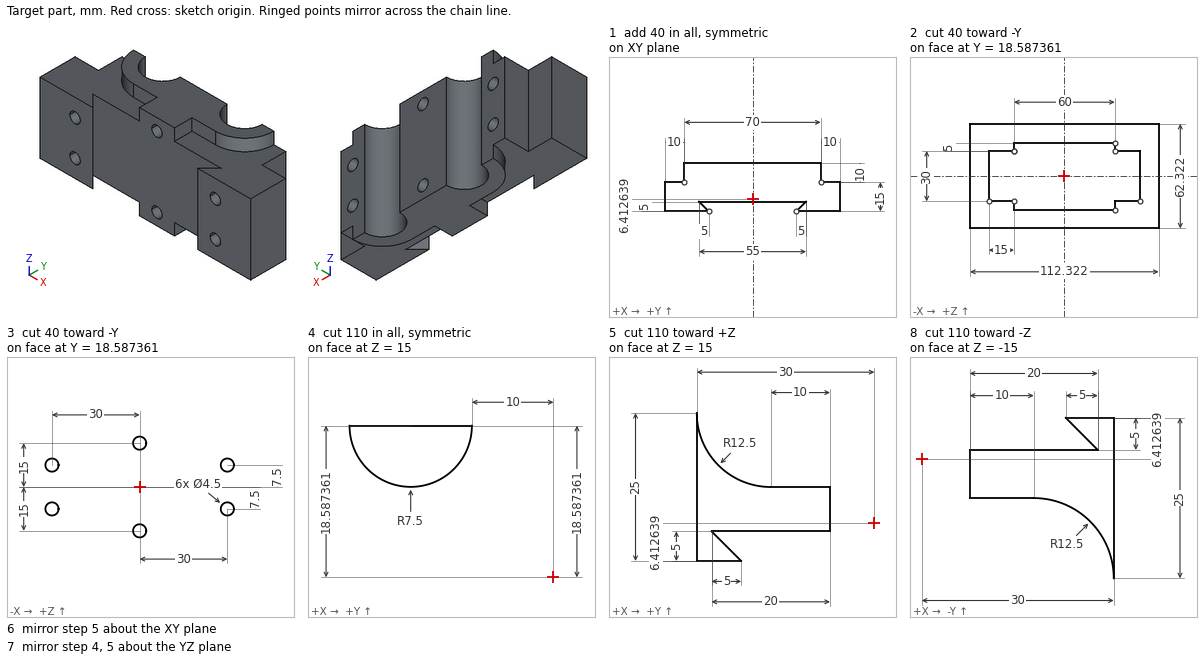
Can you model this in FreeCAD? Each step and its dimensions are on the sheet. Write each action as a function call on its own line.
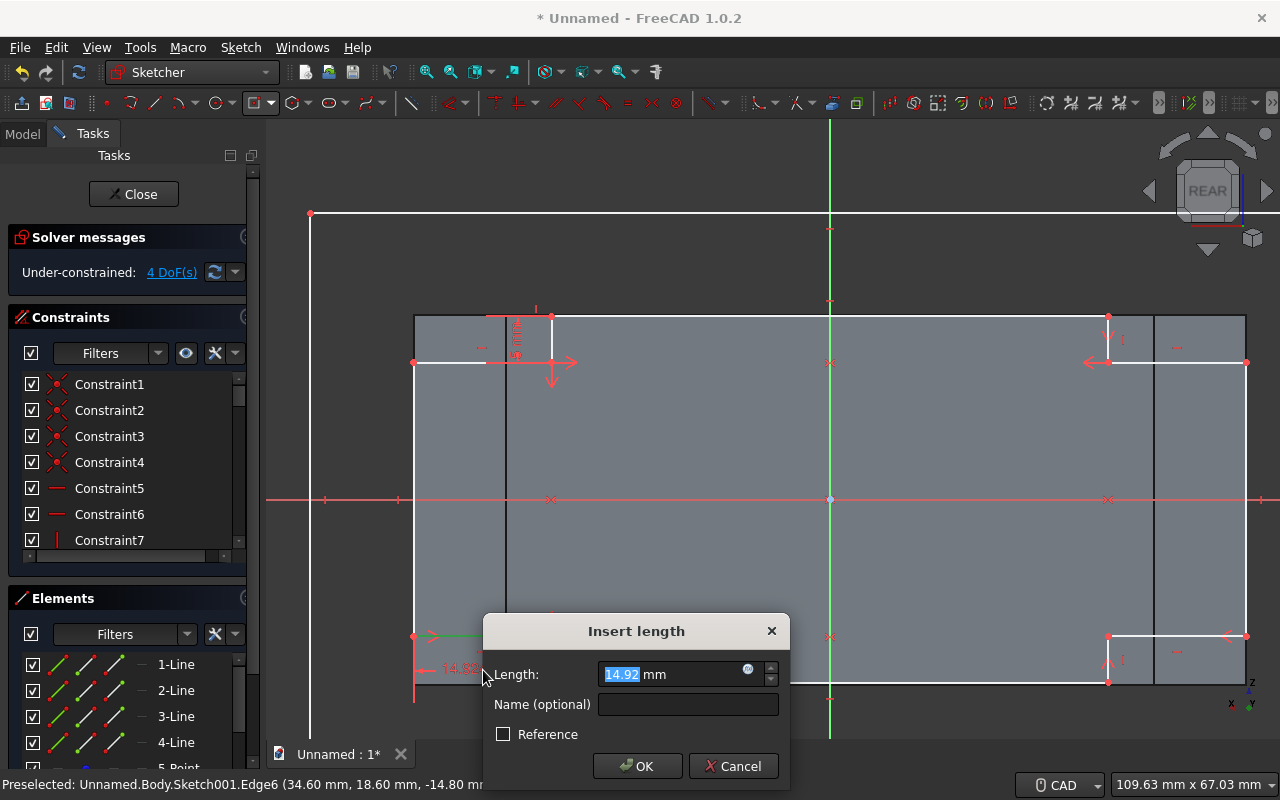
text(15)
key(Return)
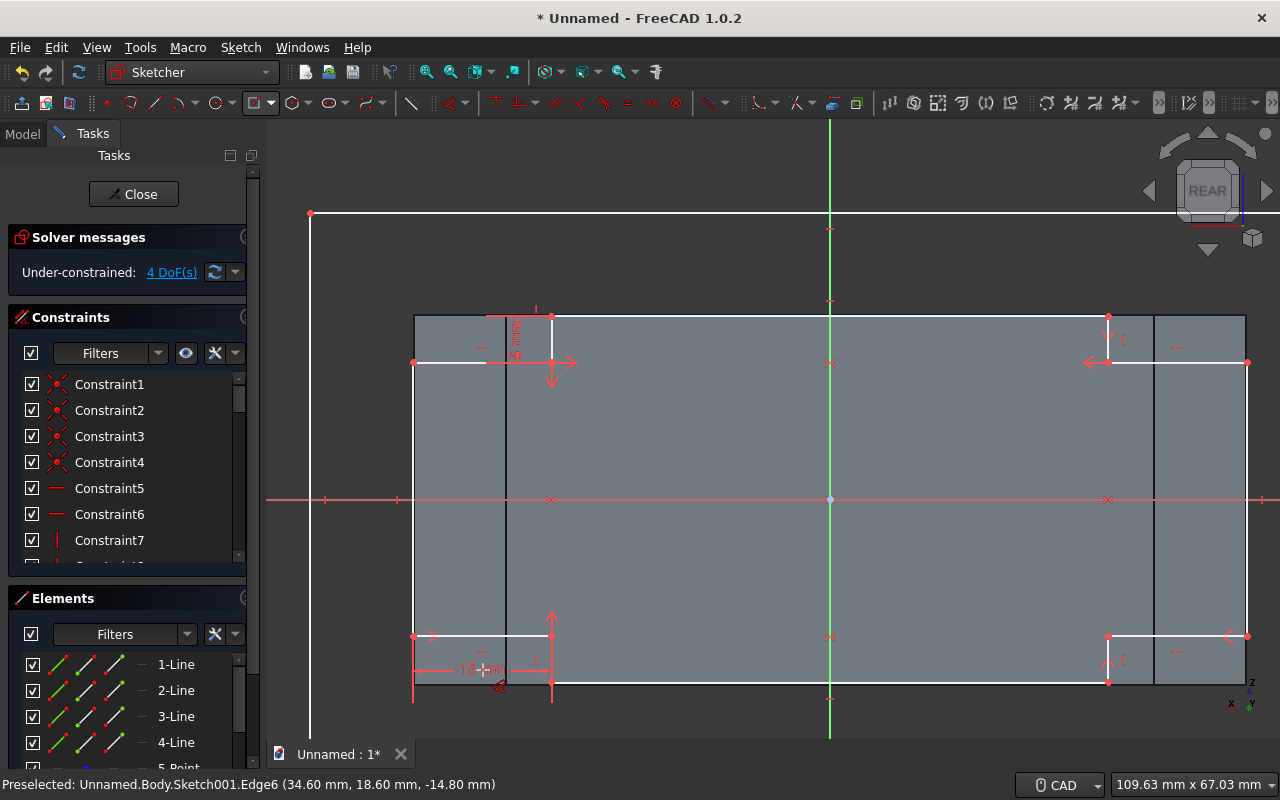
click(413, 554)
click(379, 437)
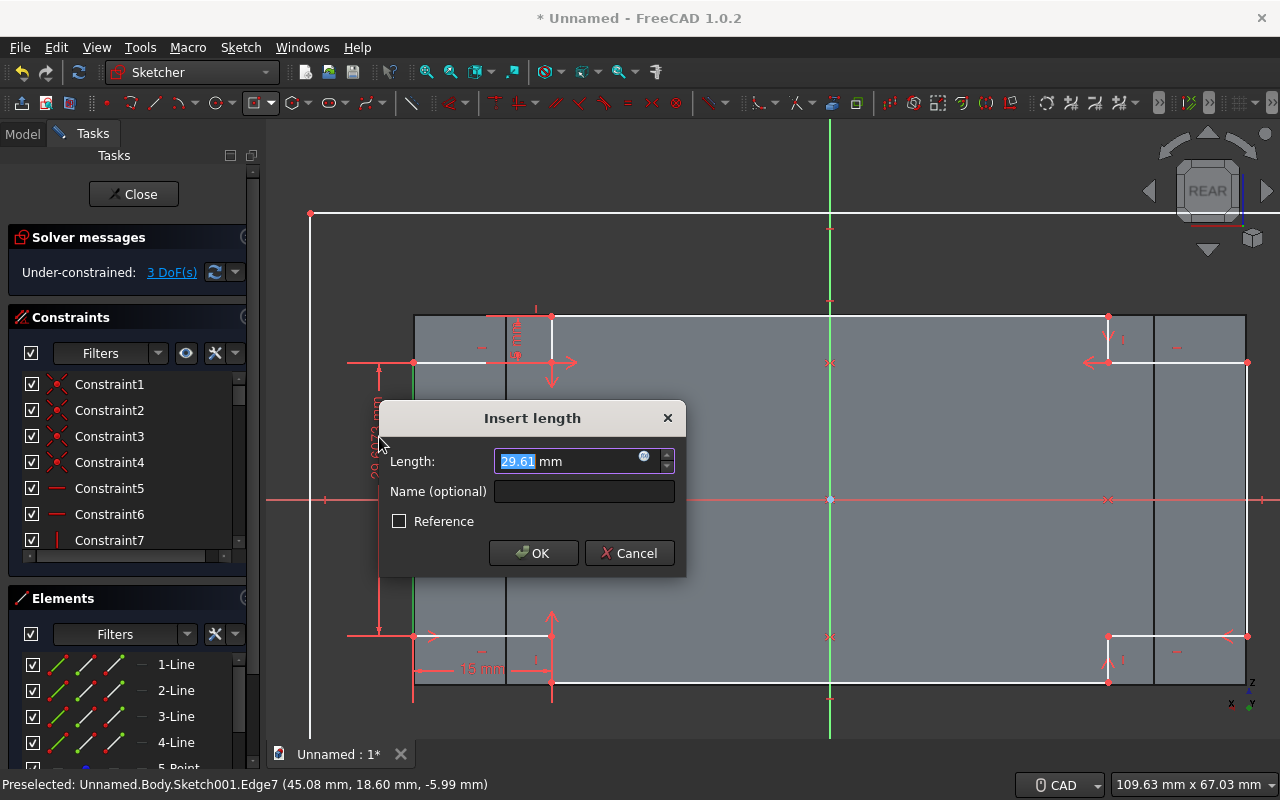
text(30)
key(Return)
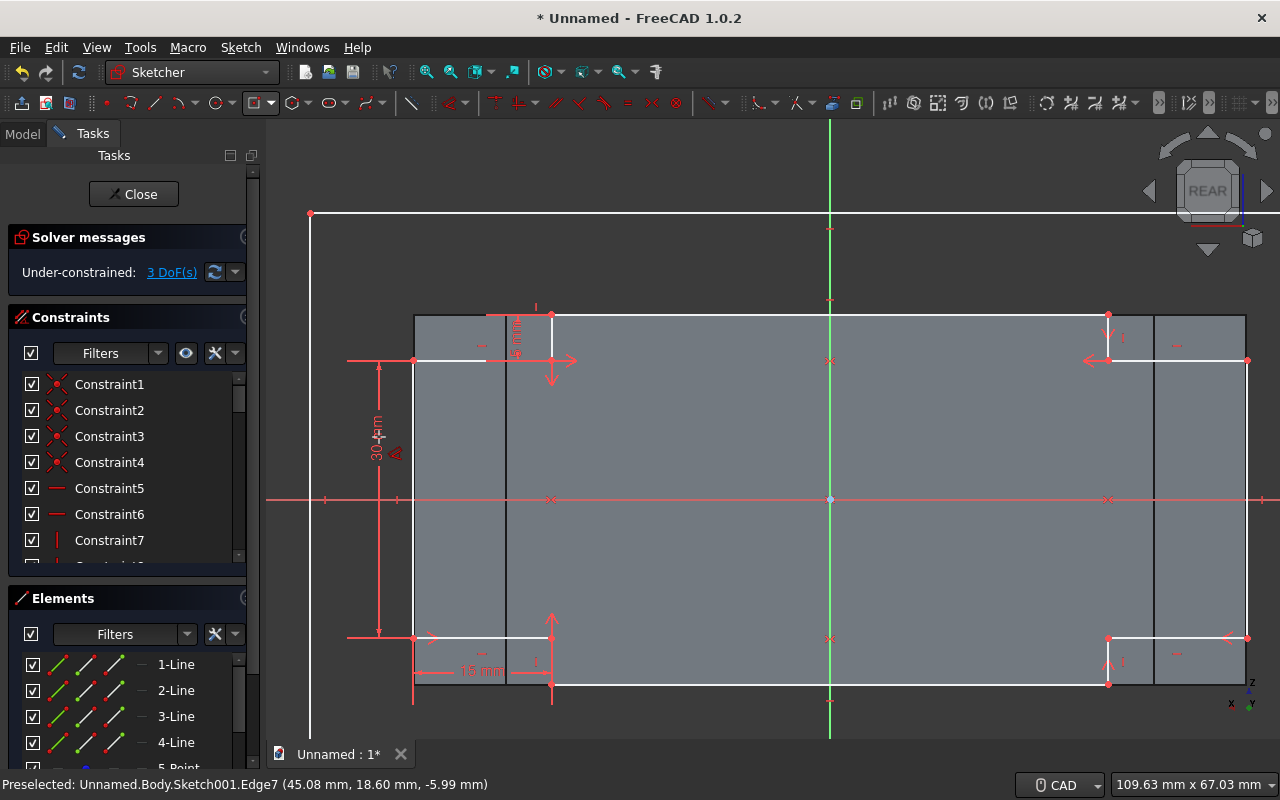
click(719, 315)
click(702, 281)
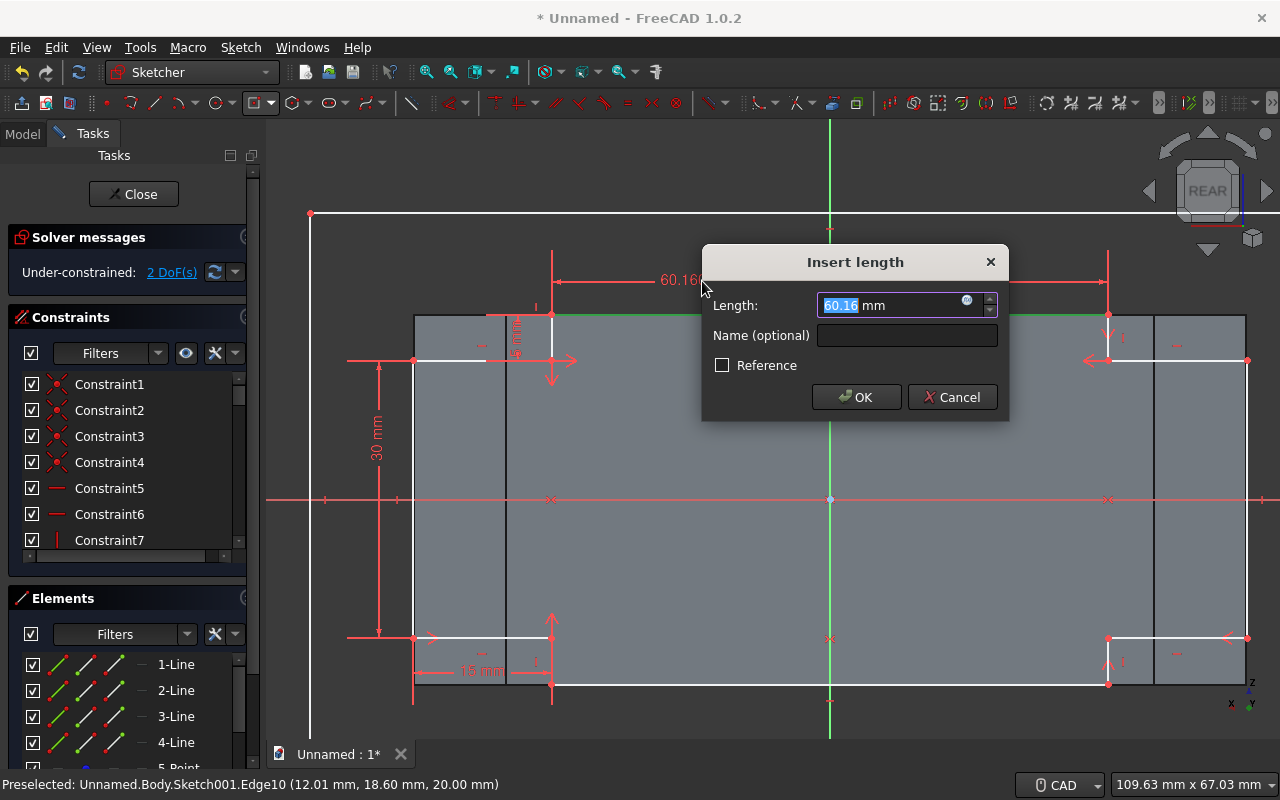
text(60)
key(Return)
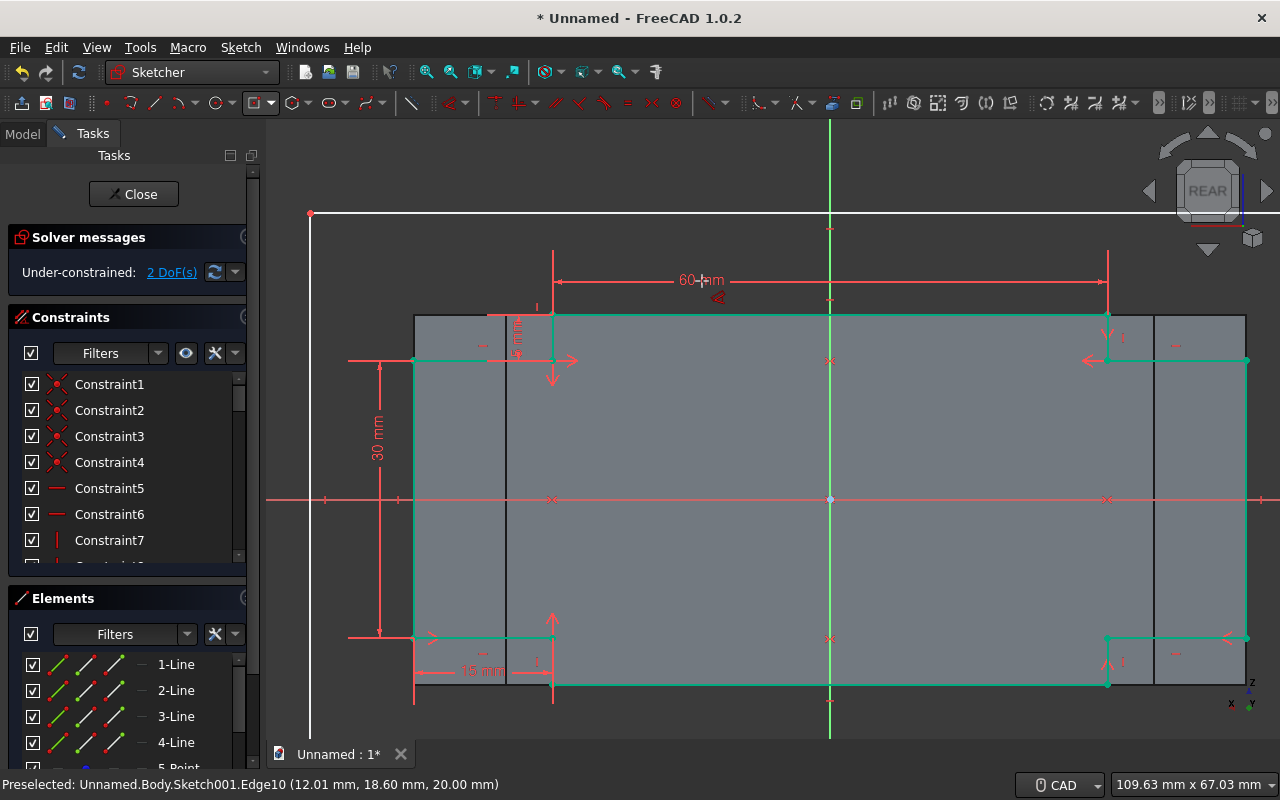
scroll(552, 343, down, 3)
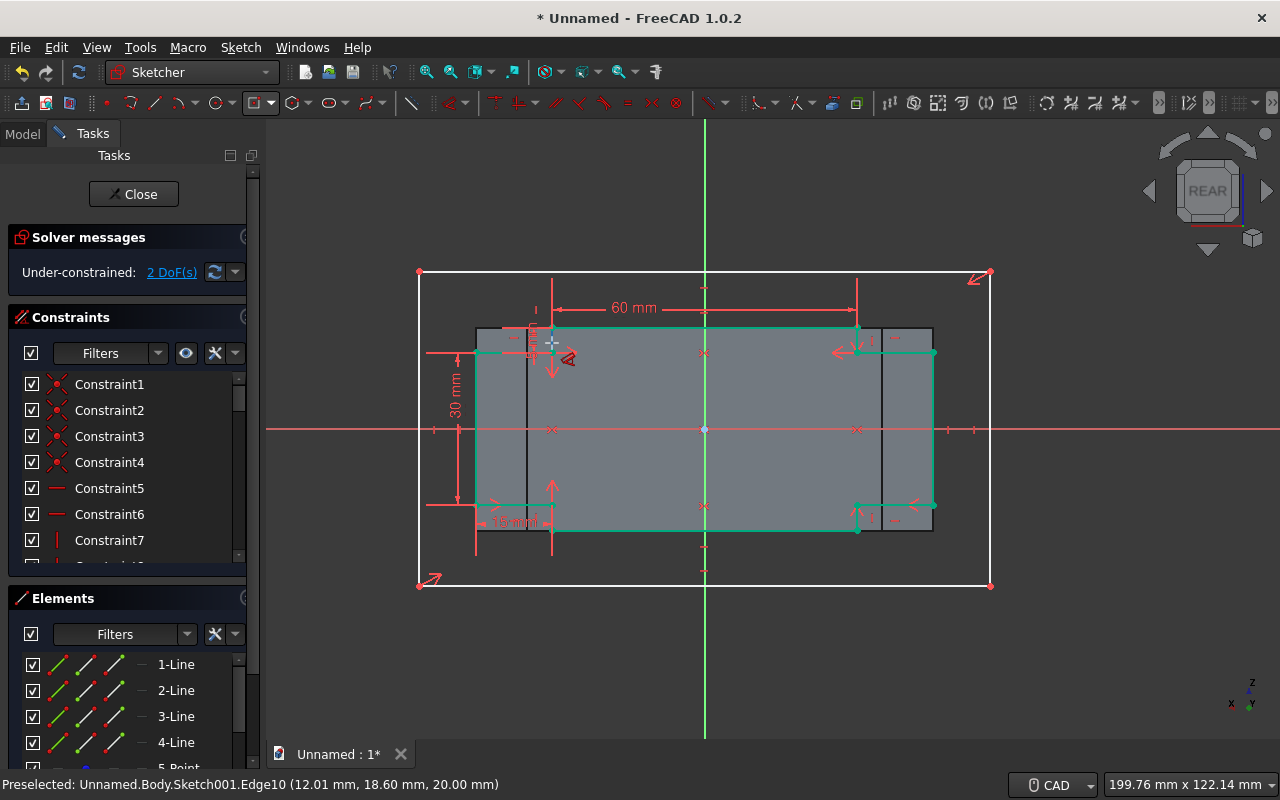
click(990, 492)
click(1024, 357)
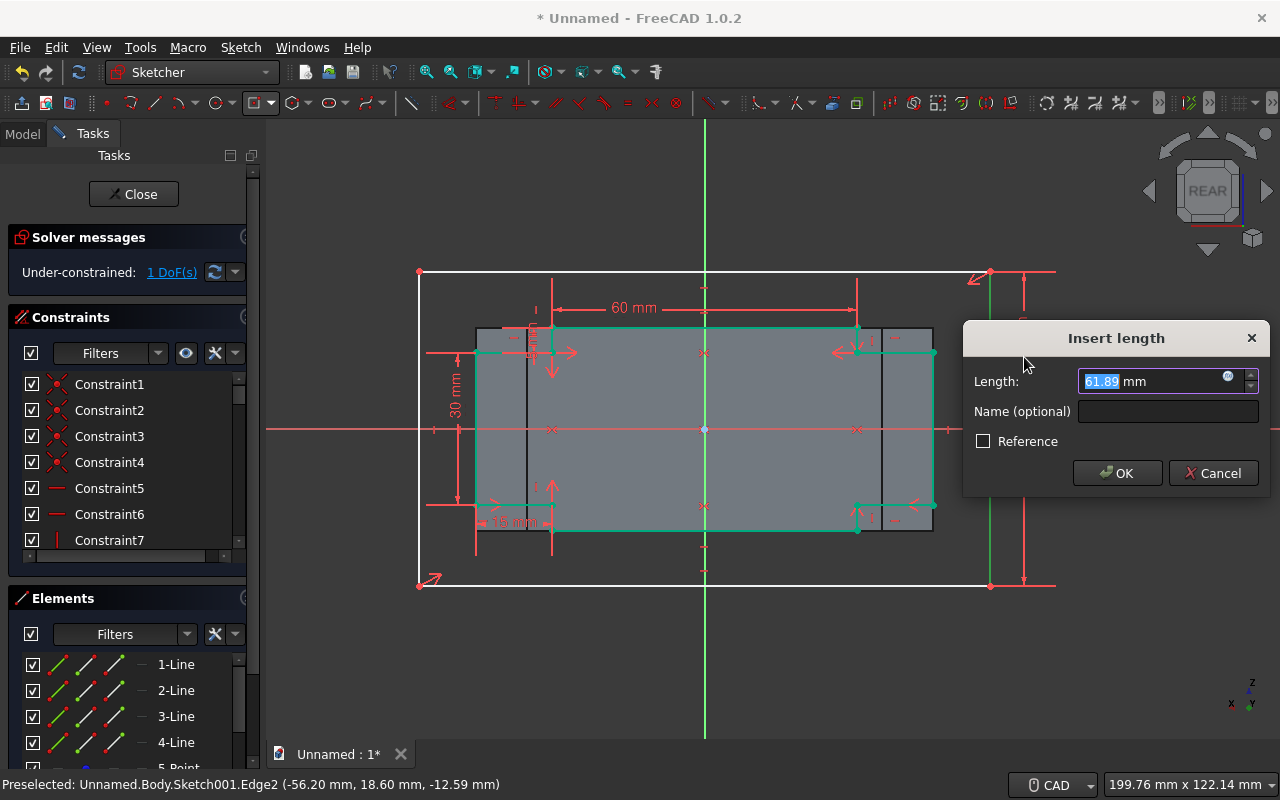
text(62.322)
key(Return)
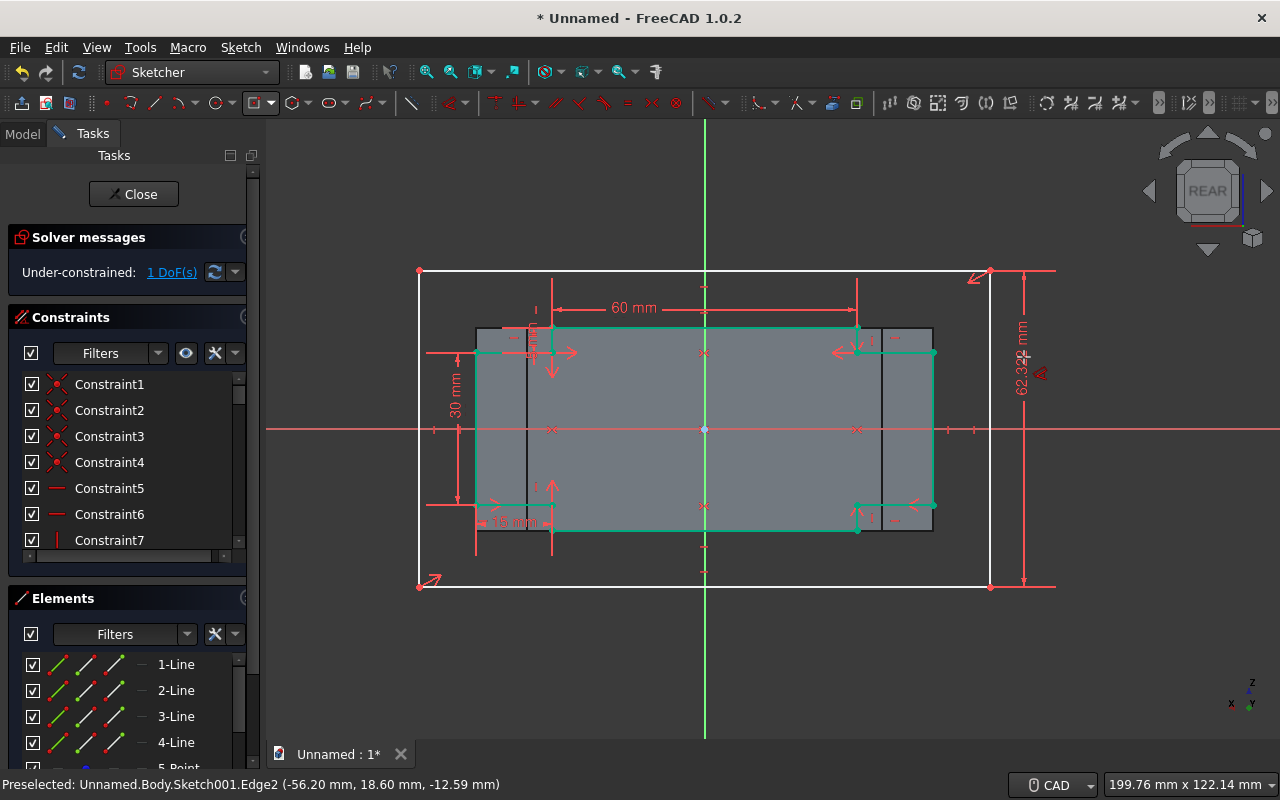
click(591, 587)
click(573, 621)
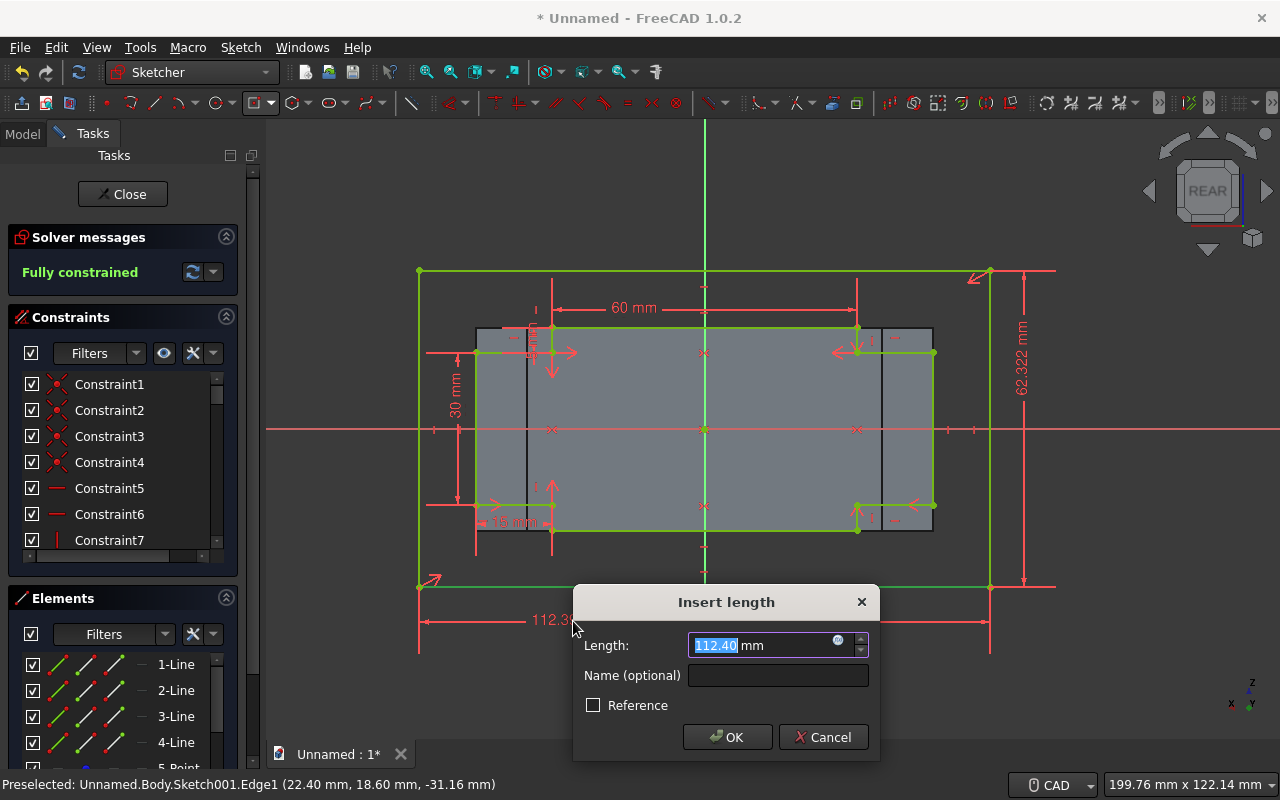
text(112.322)
key(Return)
key(Escape)